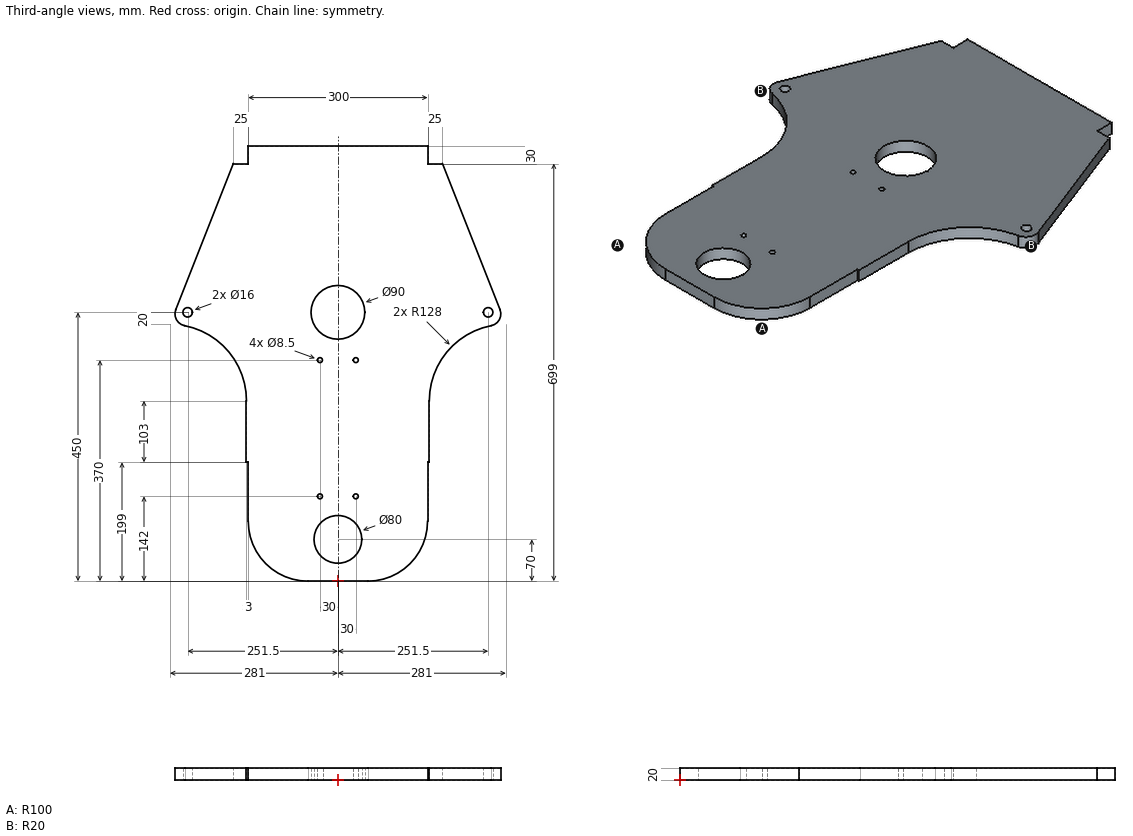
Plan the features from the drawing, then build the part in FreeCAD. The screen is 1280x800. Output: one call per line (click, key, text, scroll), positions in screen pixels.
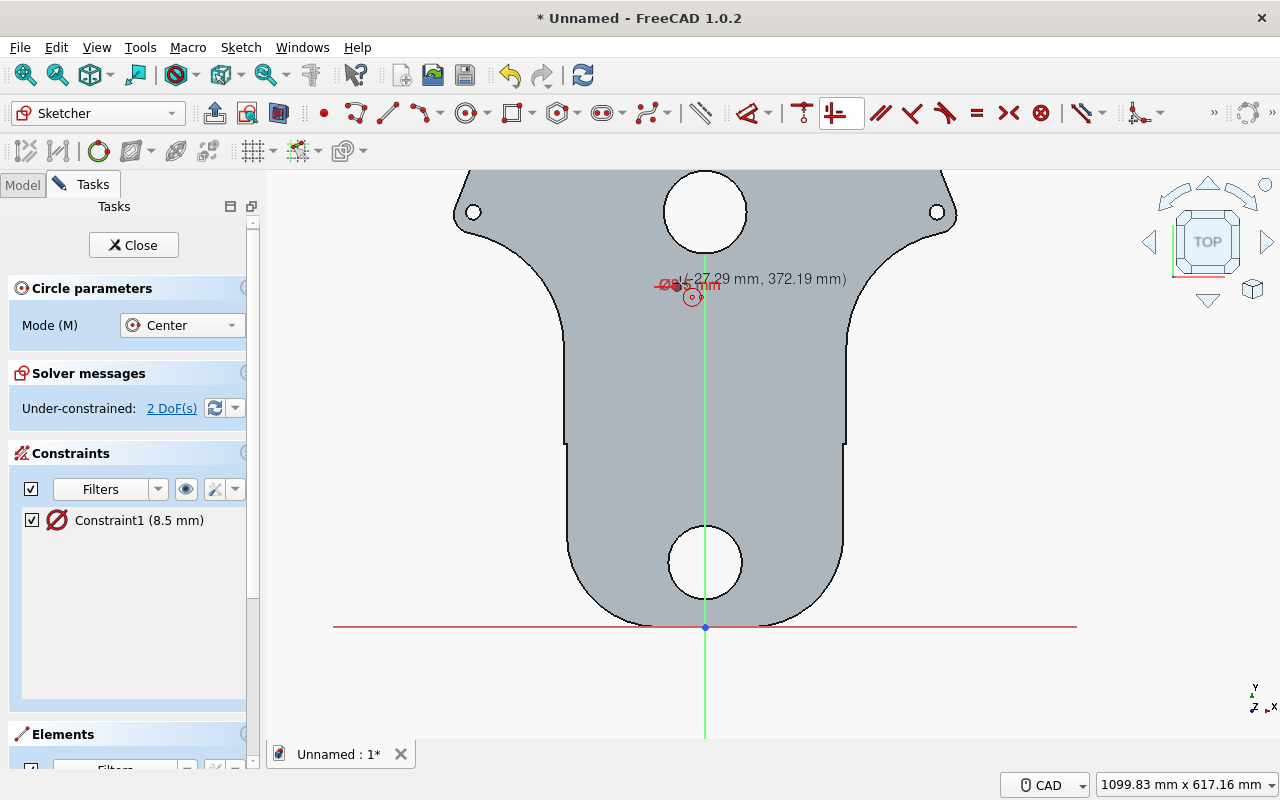
scroll(677, 496, up, 9)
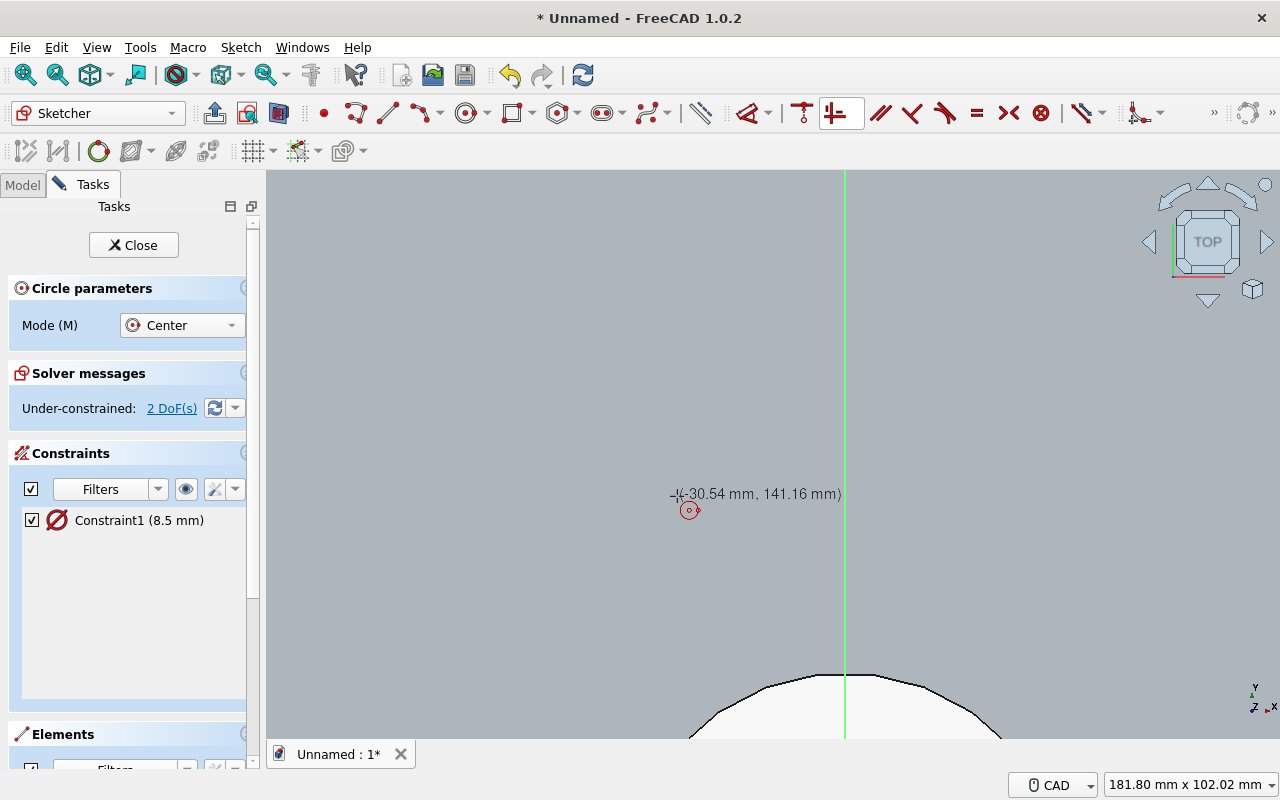
scroll(677, 496, down, 9)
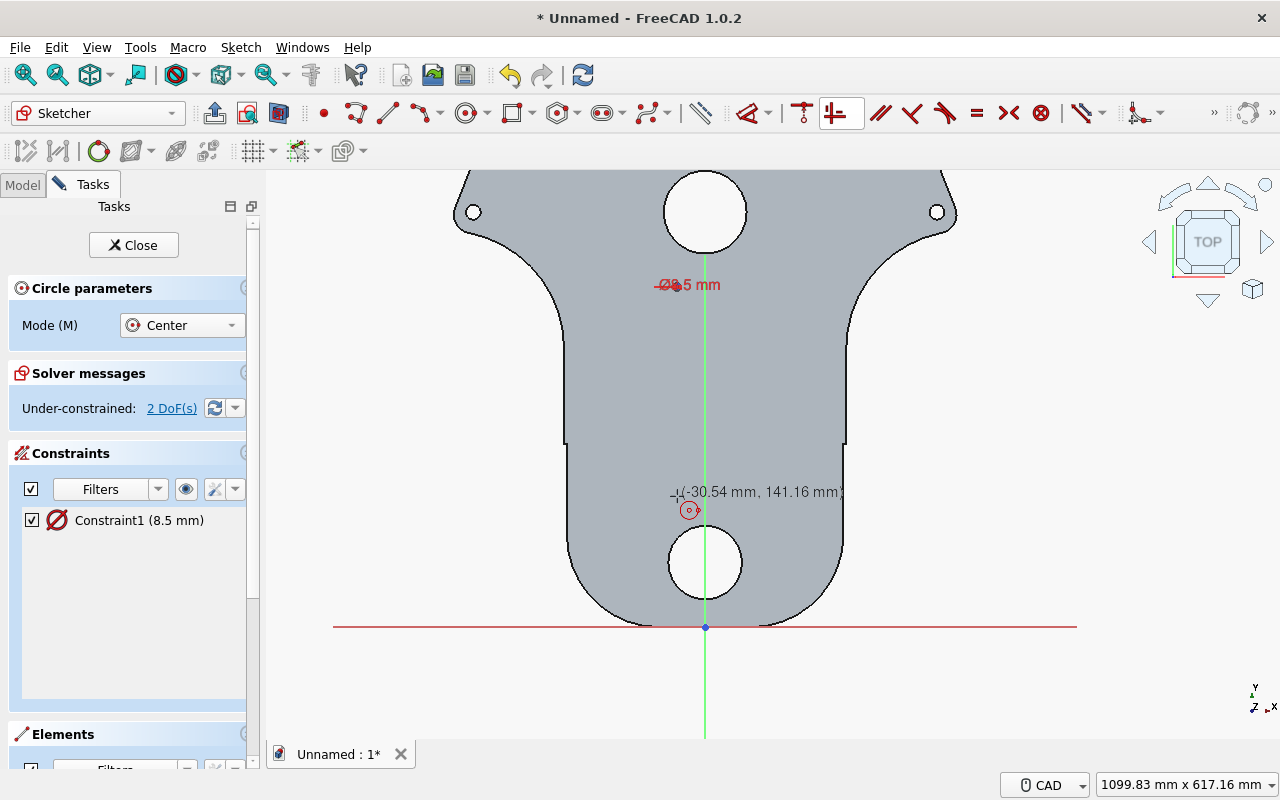
click(677, 496)
move(680, 493)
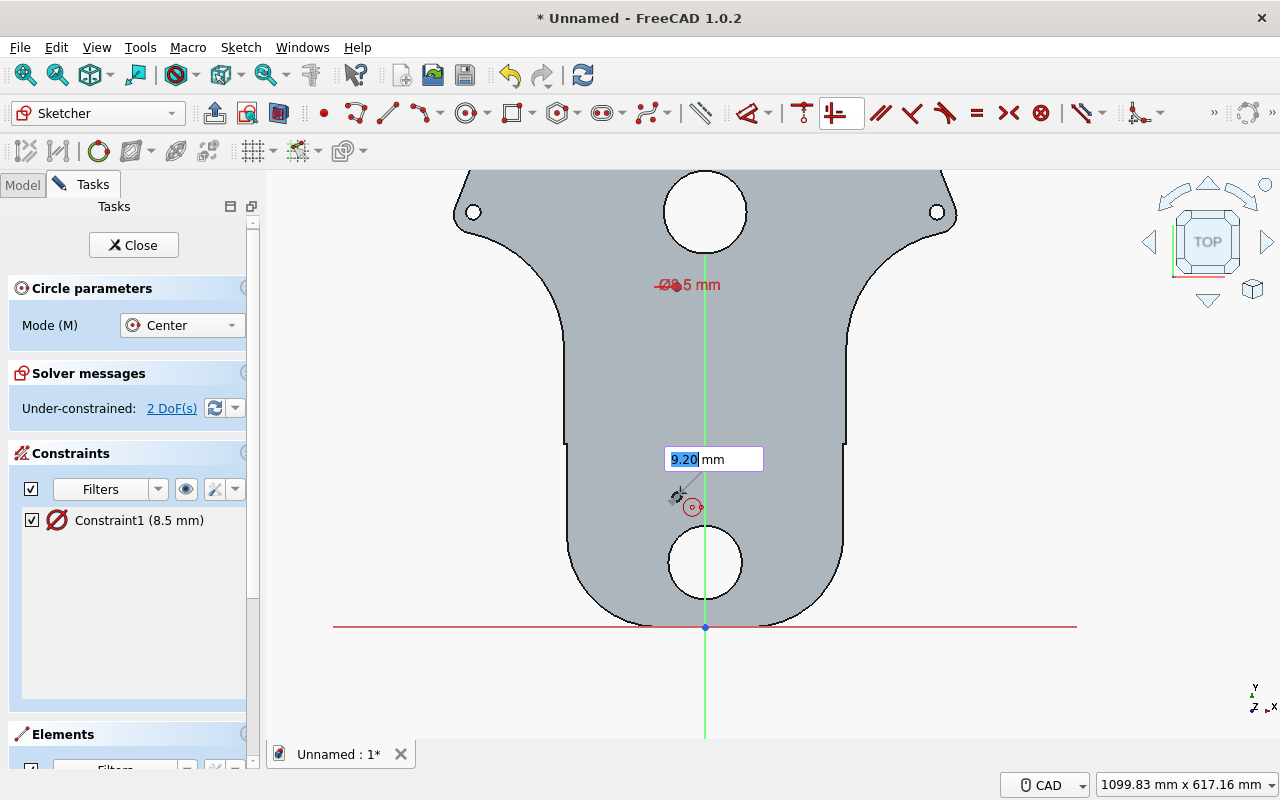
text(8.5)
key(Return)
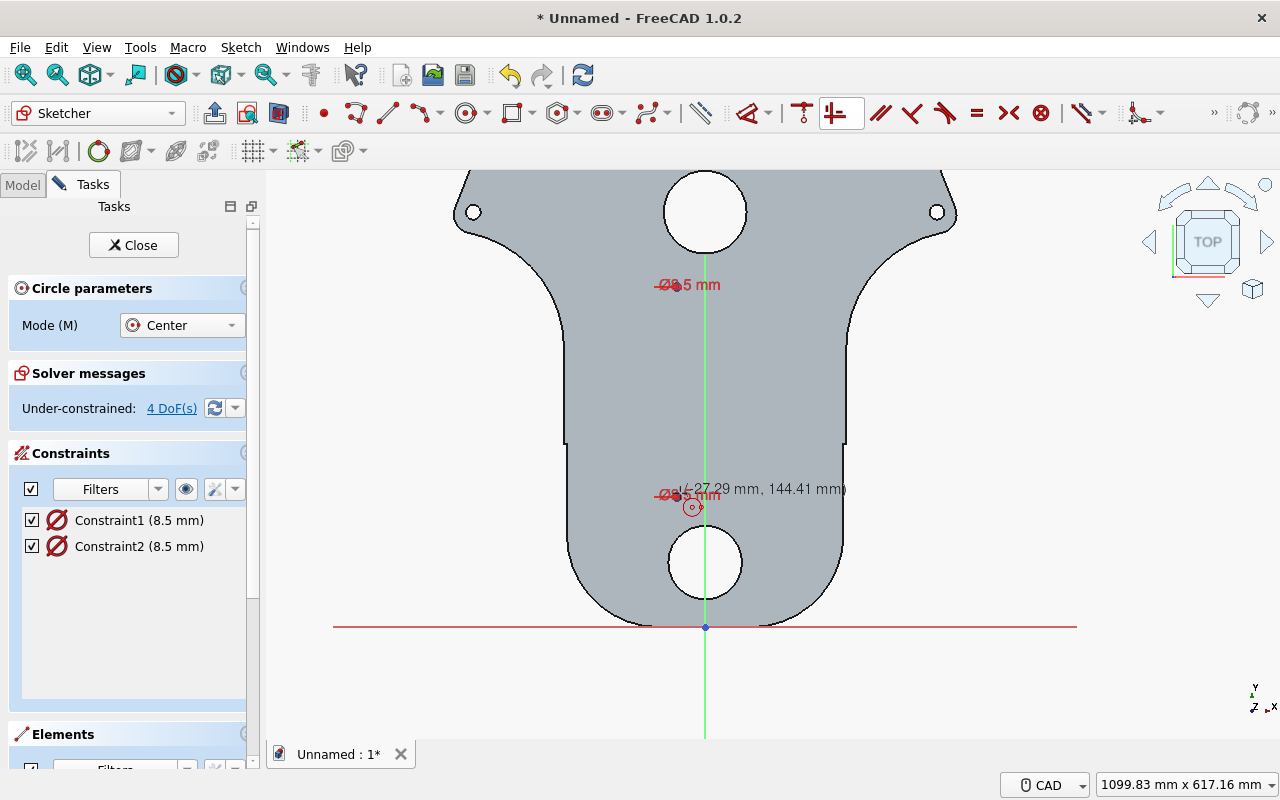
scroll(733, 496, up, 9)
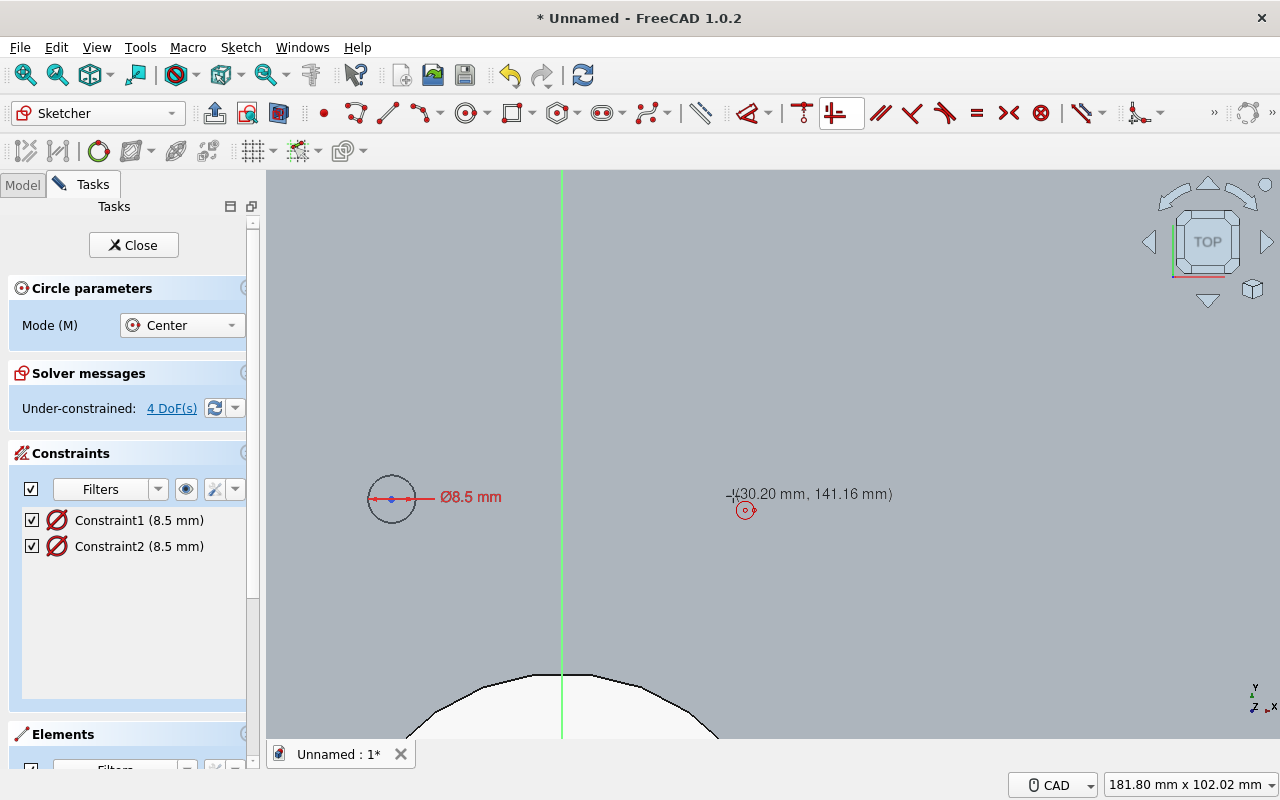
scroll(733, 496, down, 9)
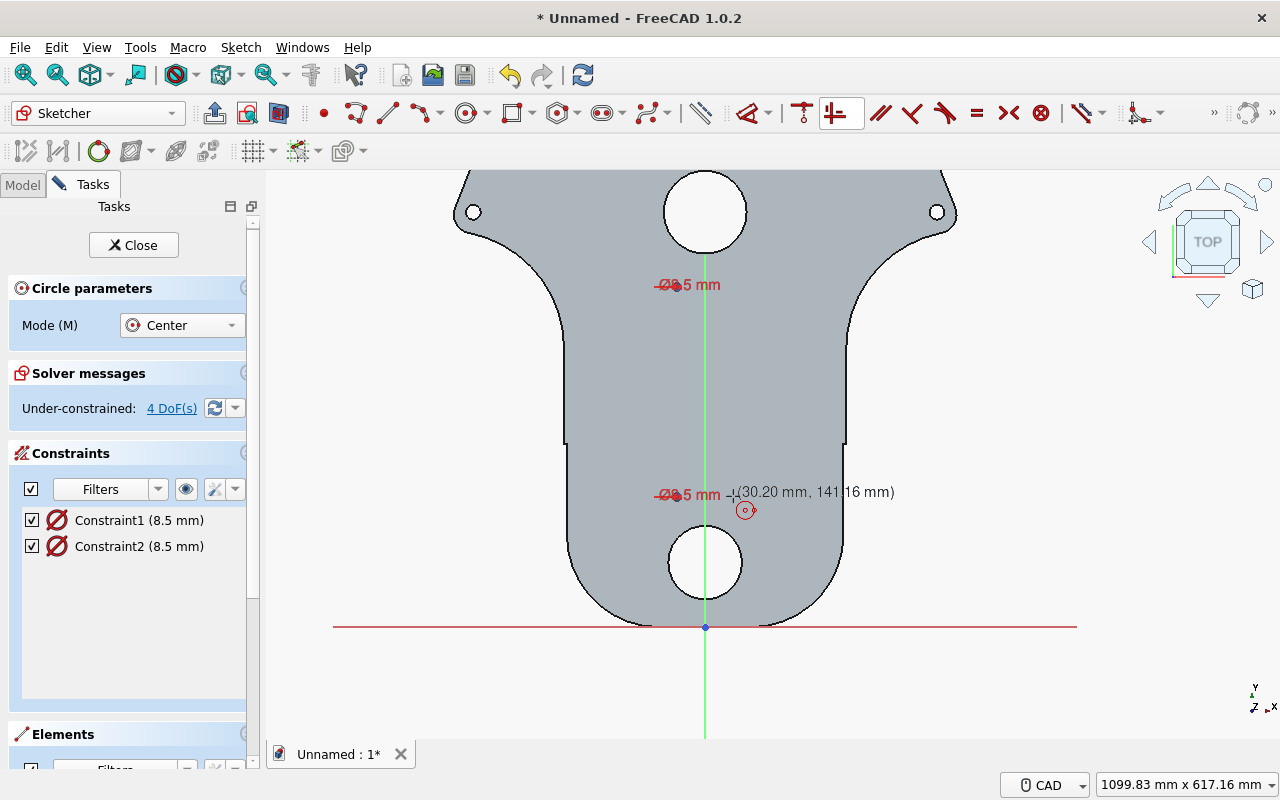
click(733, 496)
move(736, 493)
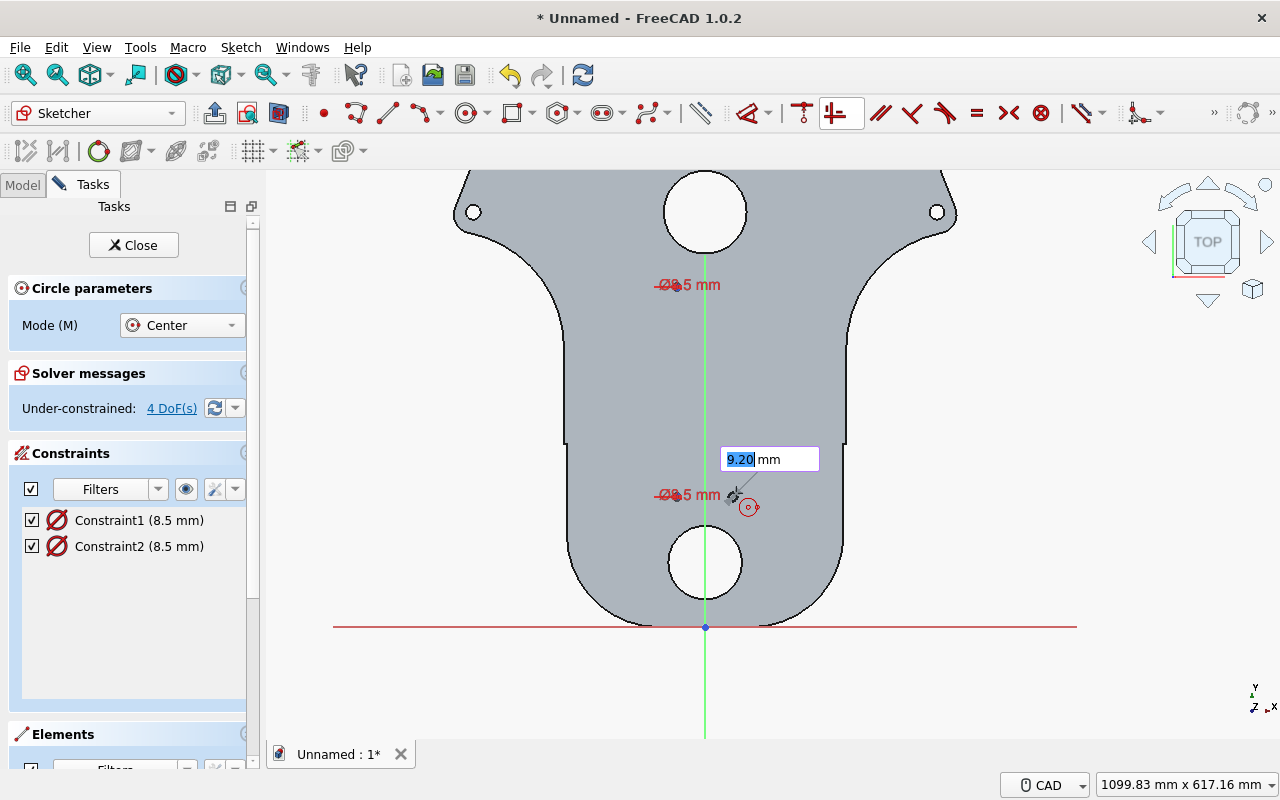
text(8.5)
key(Return)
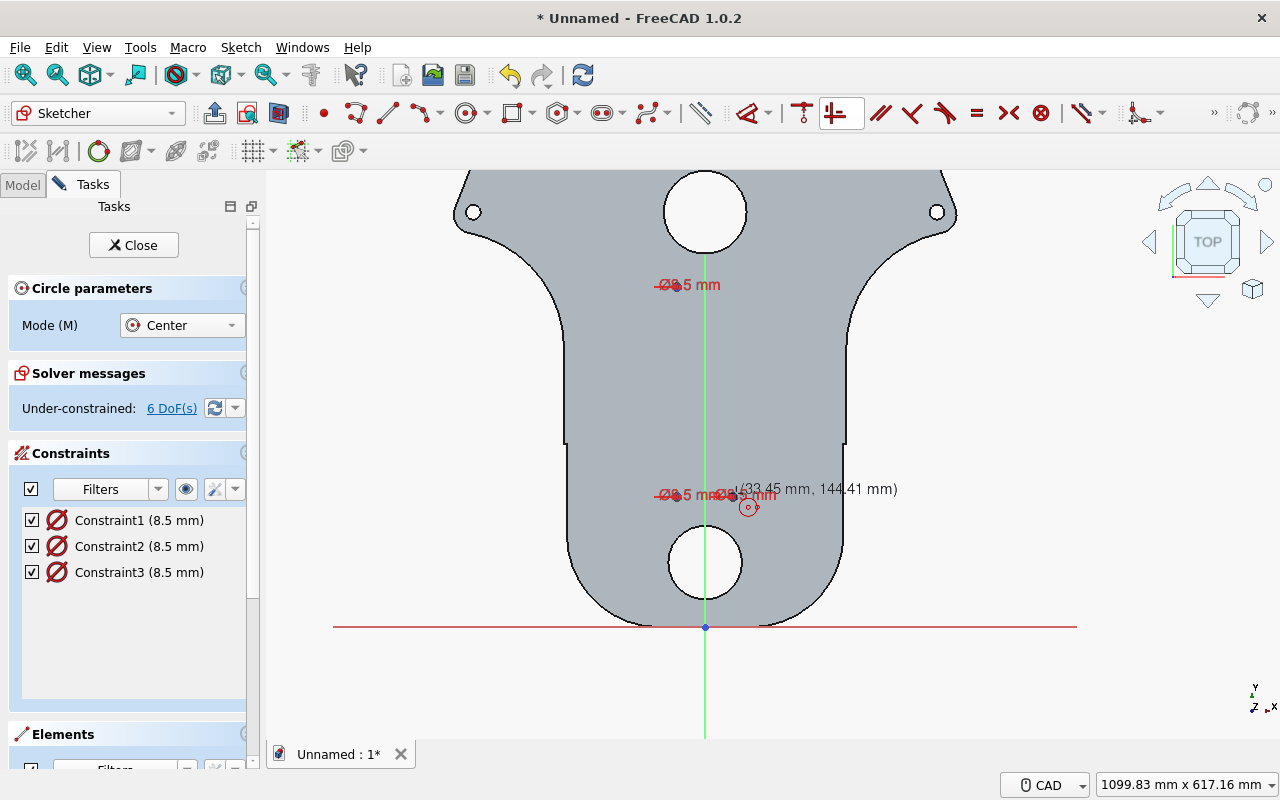
scroll(733, 286, up, 9)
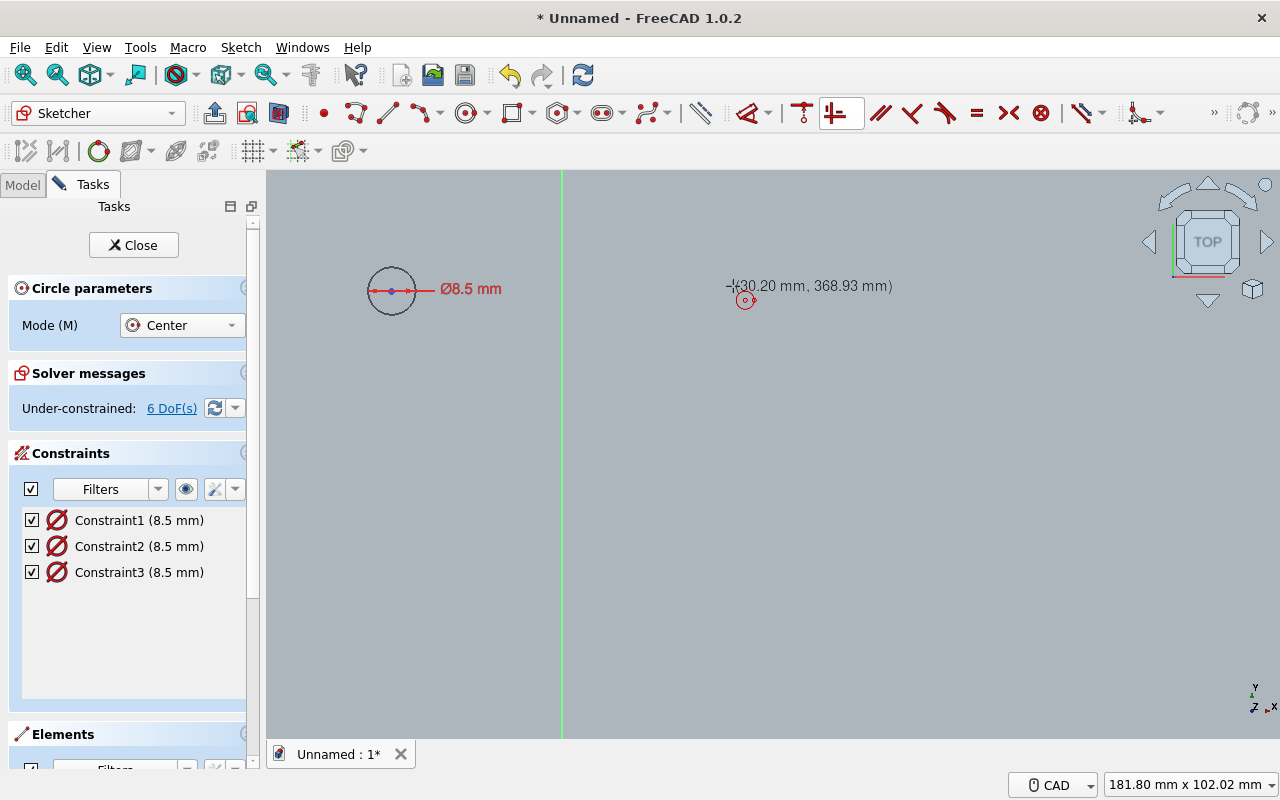
scroll(733, 286, down, 9)